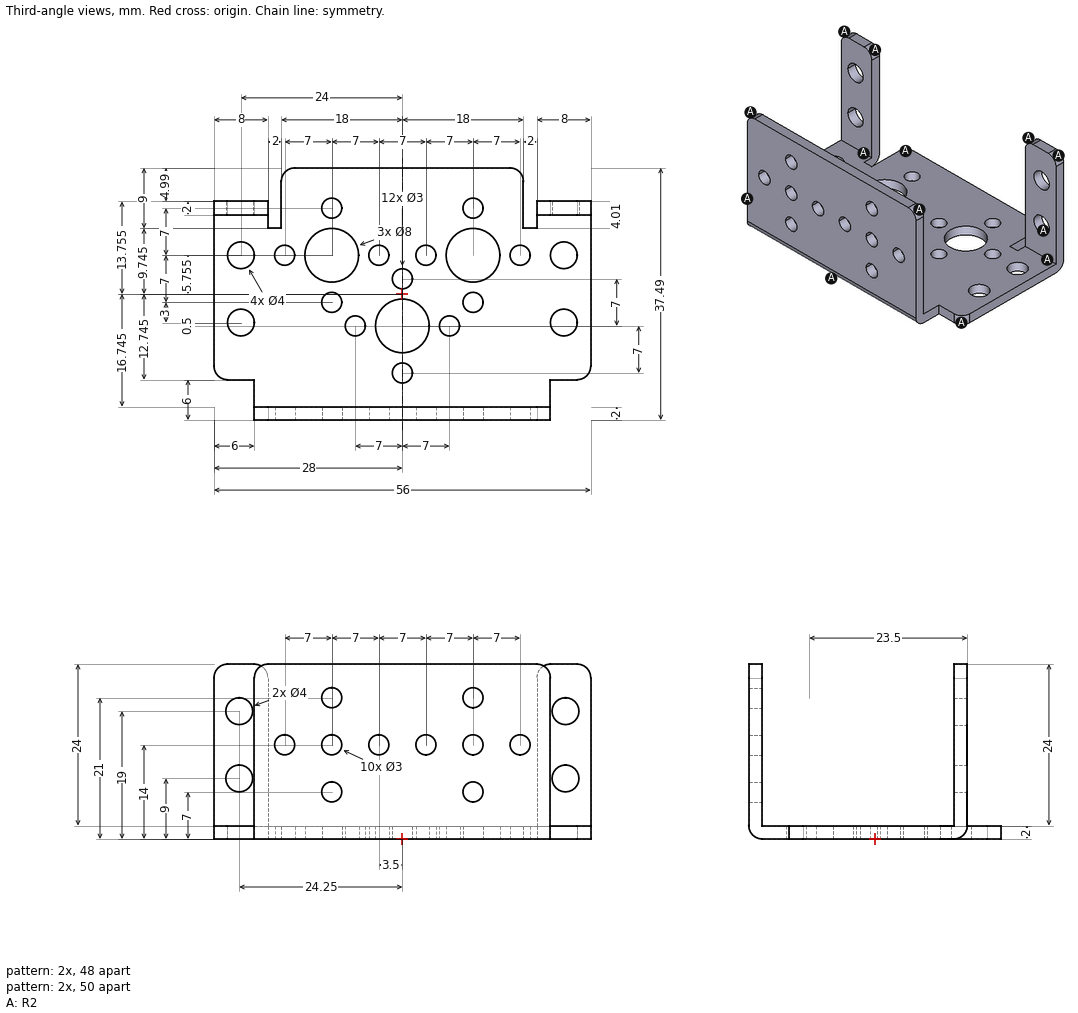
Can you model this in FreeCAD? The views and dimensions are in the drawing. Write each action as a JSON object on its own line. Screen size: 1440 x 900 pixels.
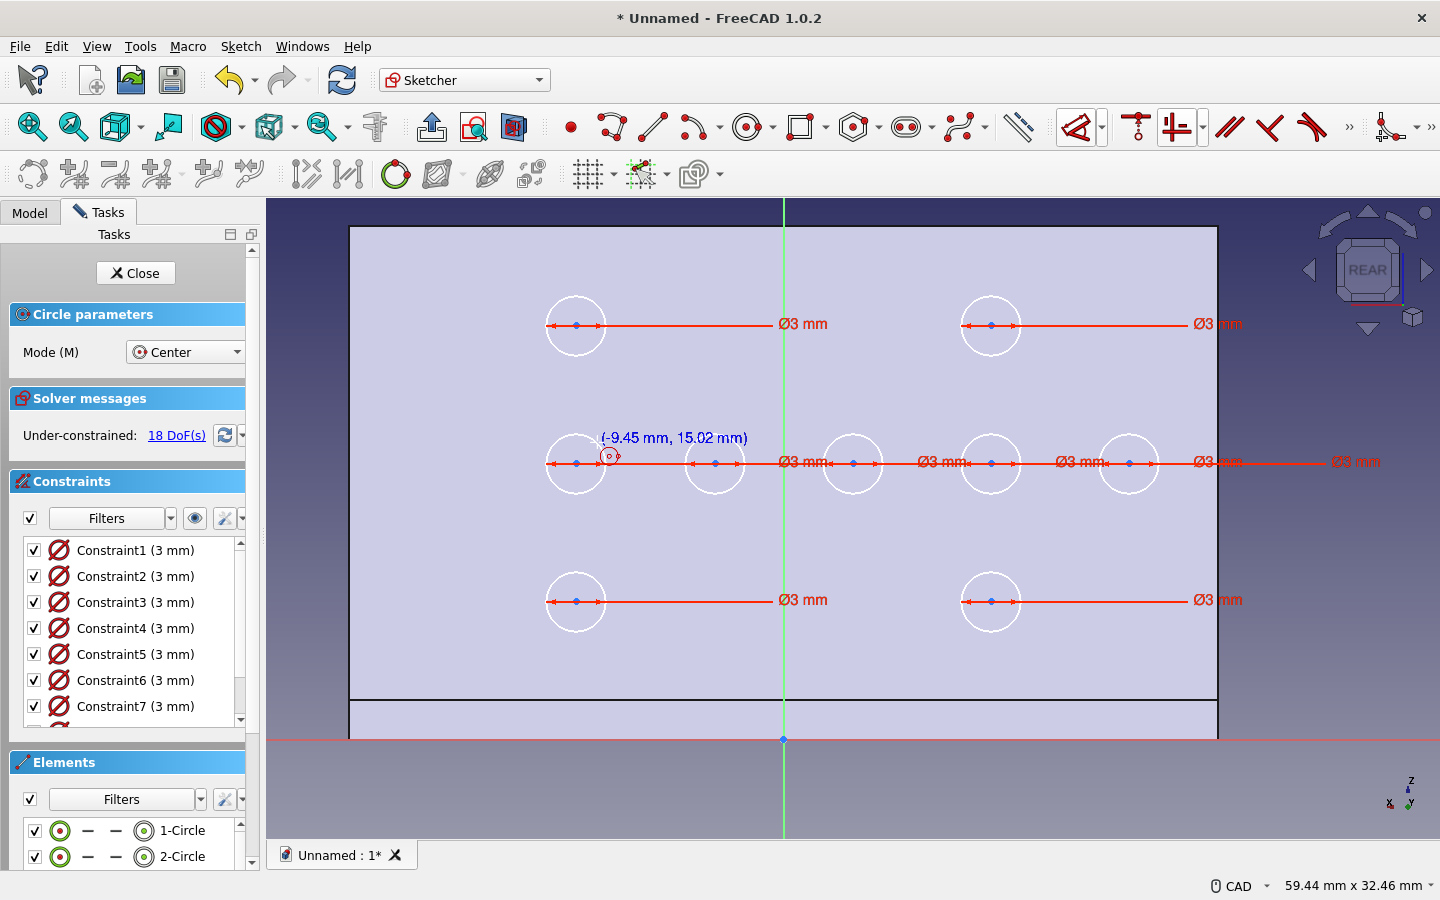
{"action": "left_click", "coordinate": [438, 463]}
{"action": "mouse_move", "coordinate": [459, 442]}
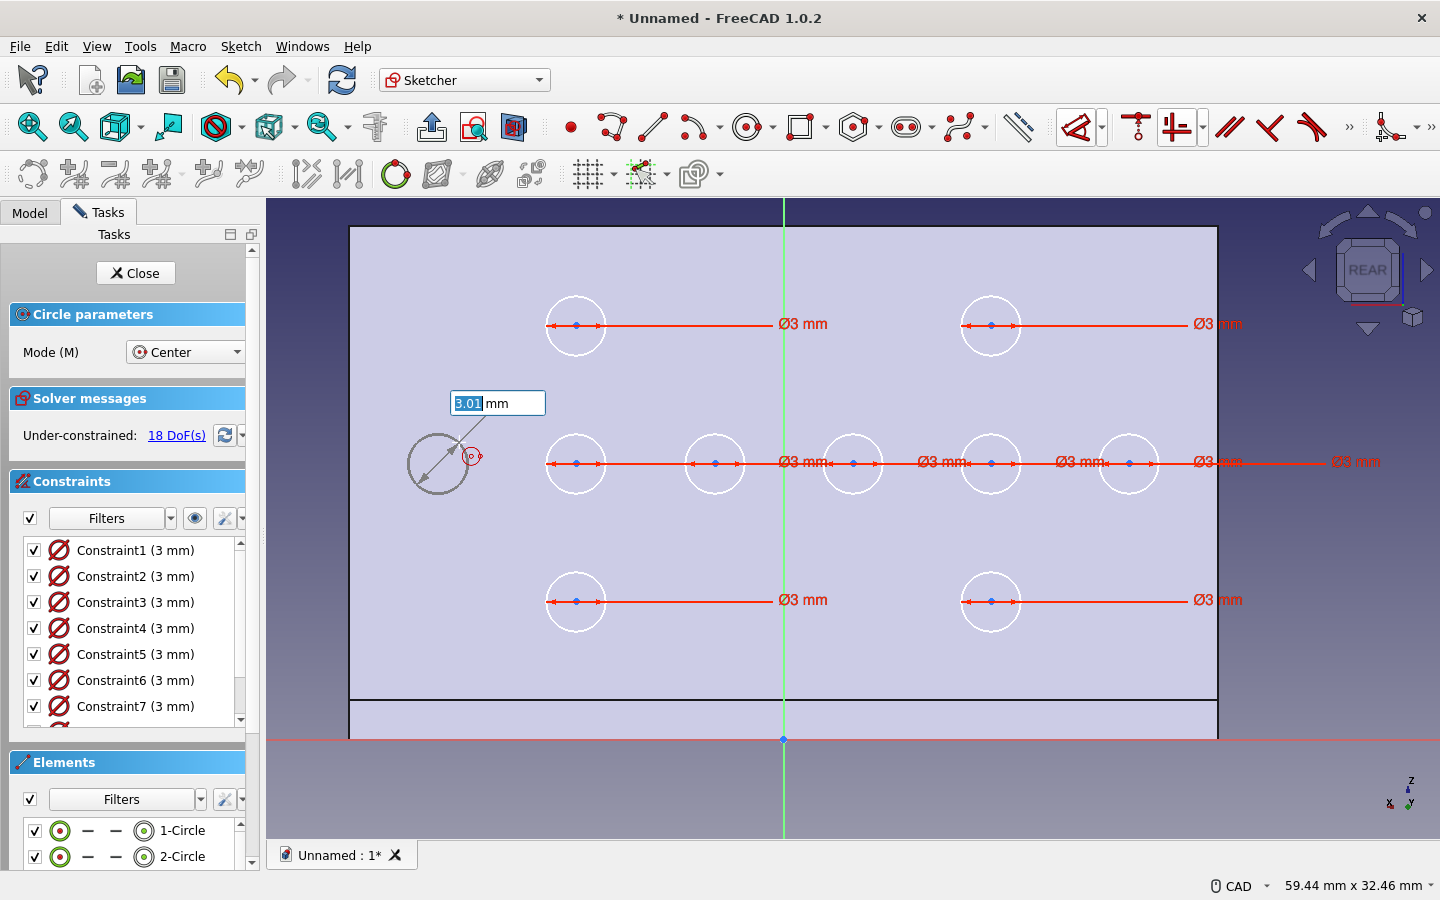
{"action": "type", "text": "3"}
{"action": "key", "text": "Return"}
{"action": "key", "text": "Escape"}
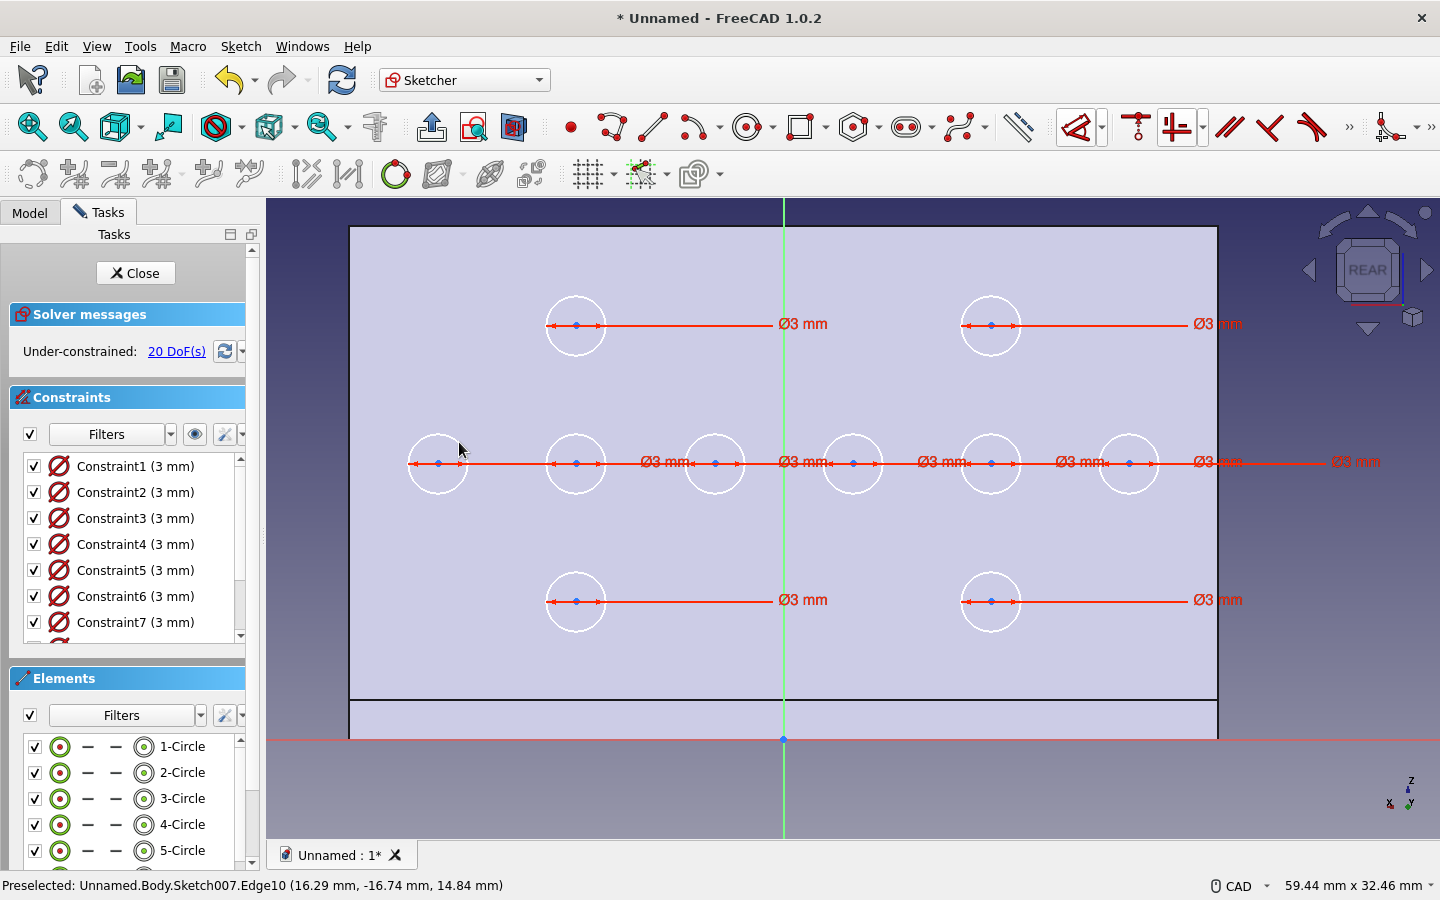
{"action": "left_click", "coordinate": [991, 464]}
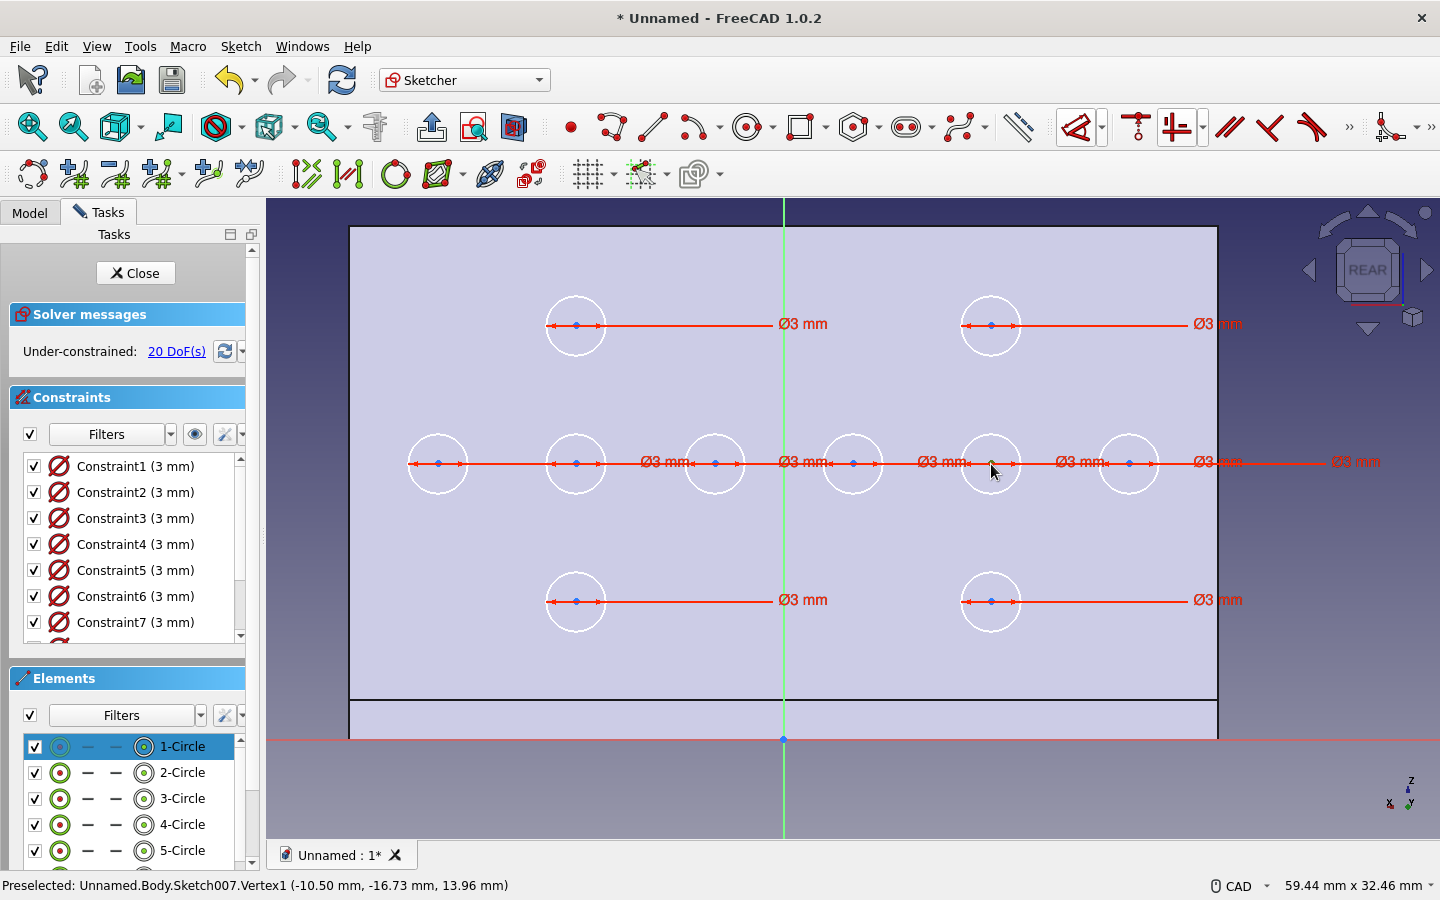
{"action": "left_click", "coordinate": [1129, 464]}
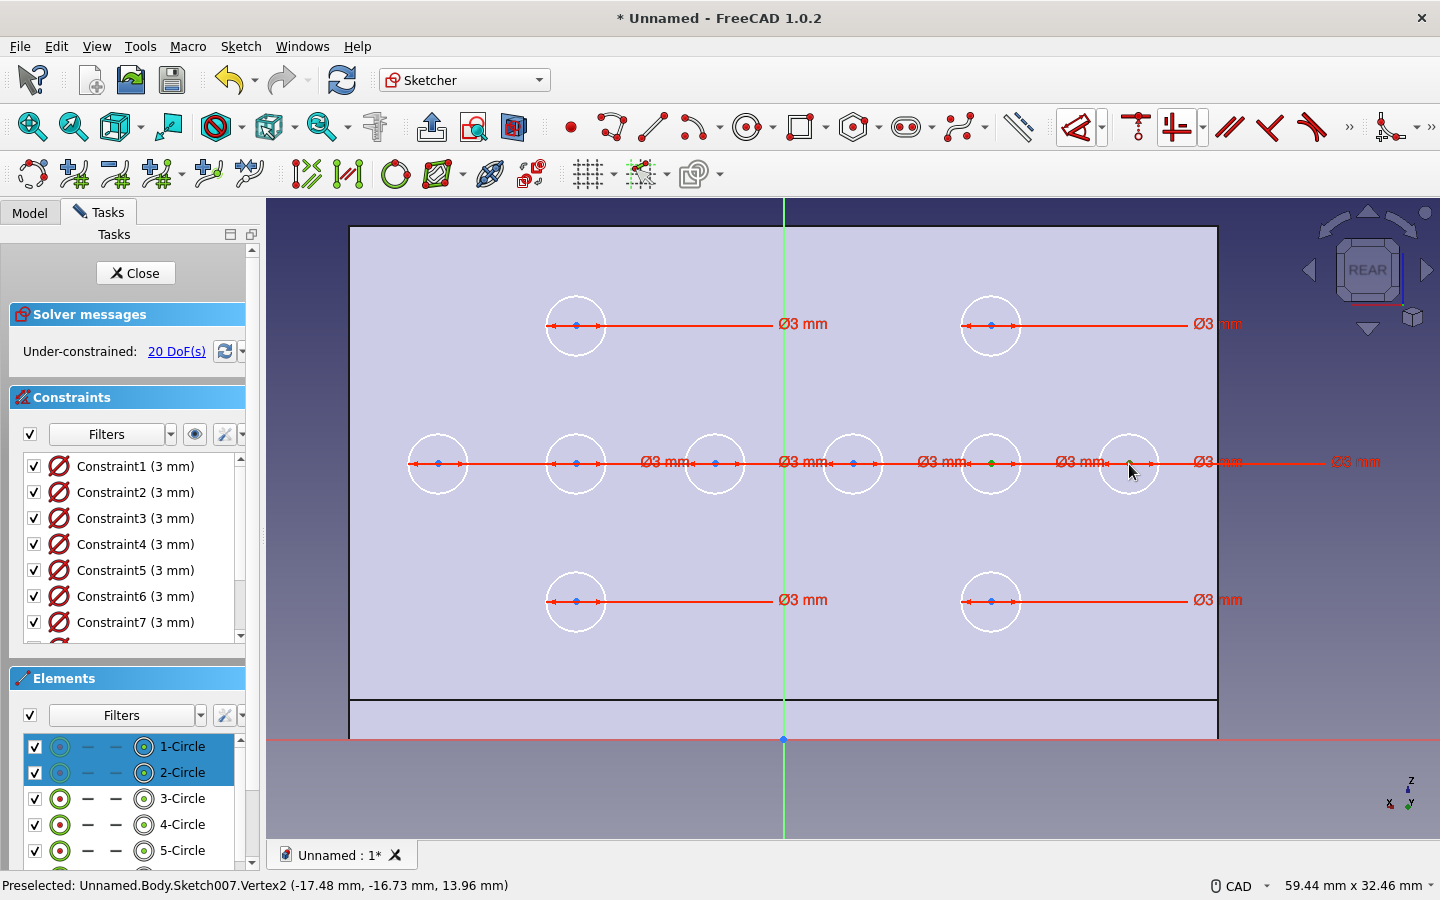
{"action": "key", "text": "h"}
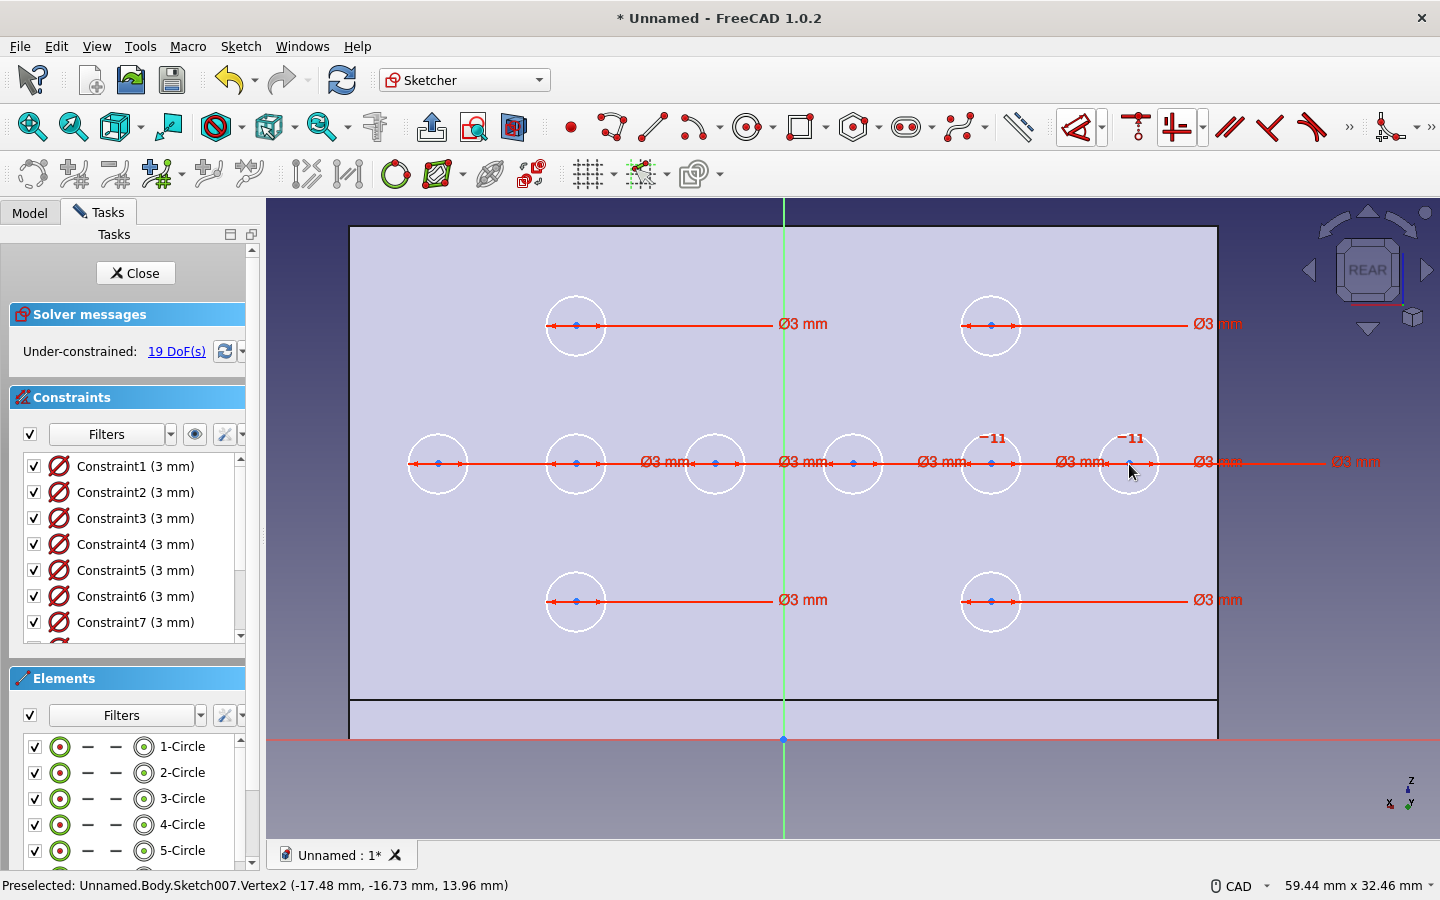
{"action": "left_click", "coordinate": [991, 464]}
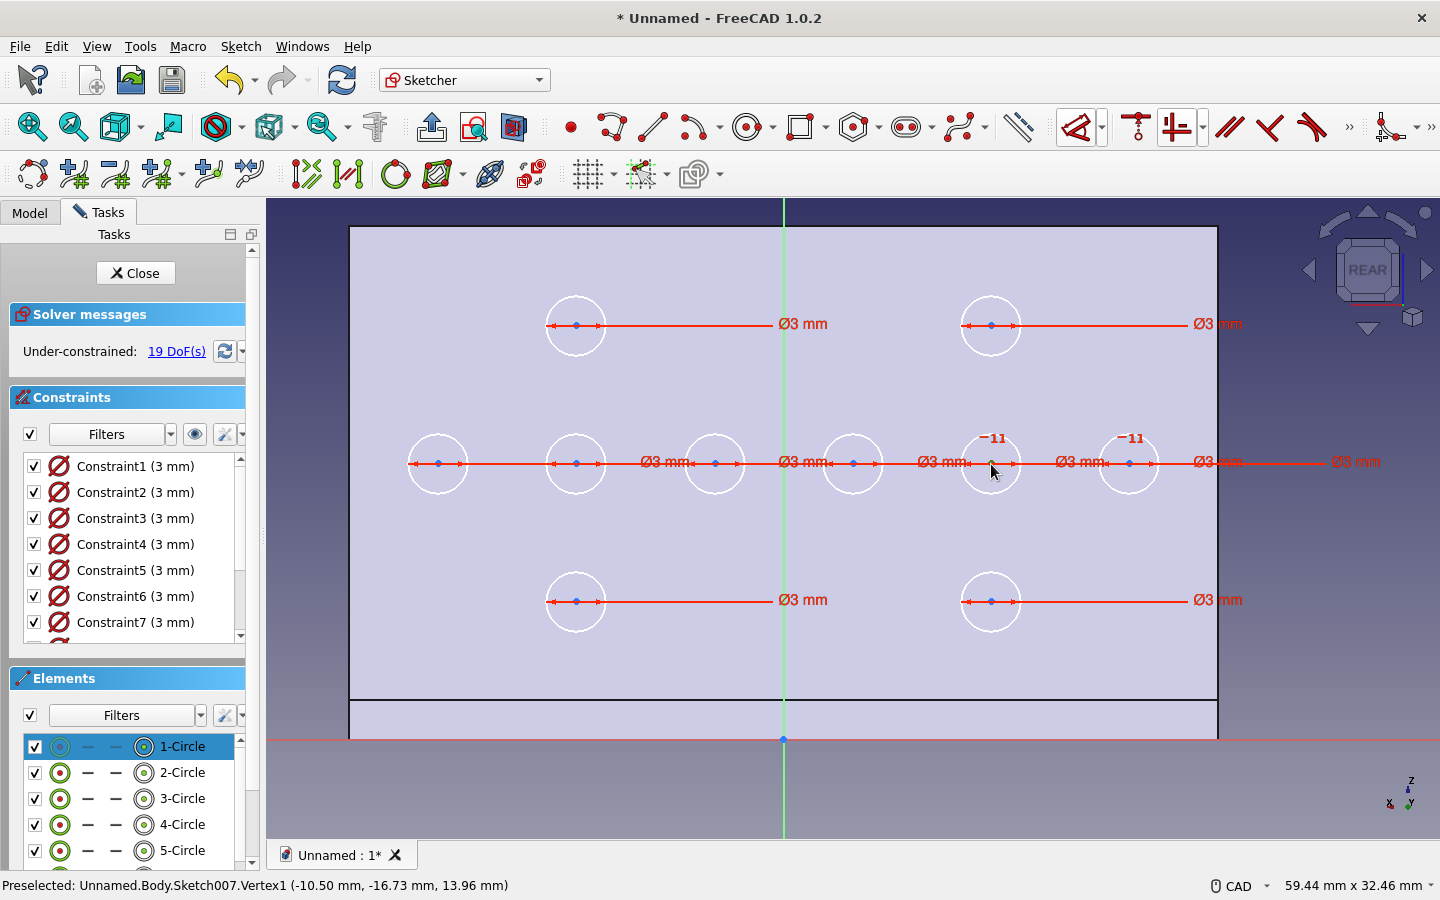
{"action": "left_click", "coordinate": [991, 326]}